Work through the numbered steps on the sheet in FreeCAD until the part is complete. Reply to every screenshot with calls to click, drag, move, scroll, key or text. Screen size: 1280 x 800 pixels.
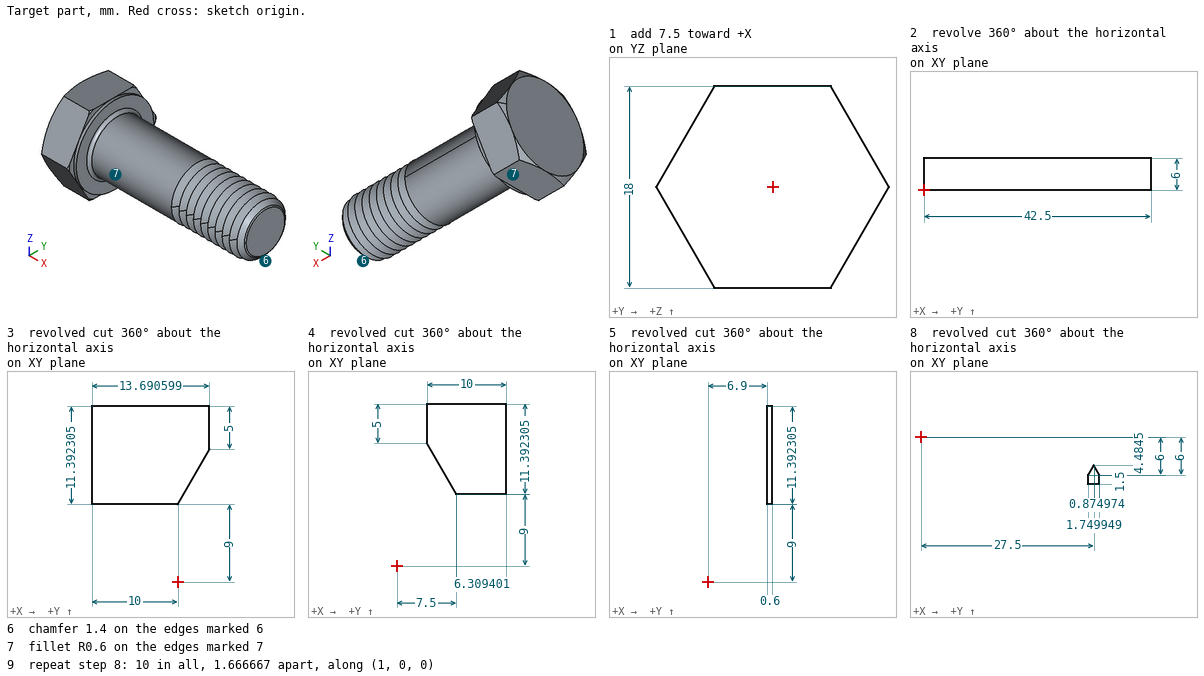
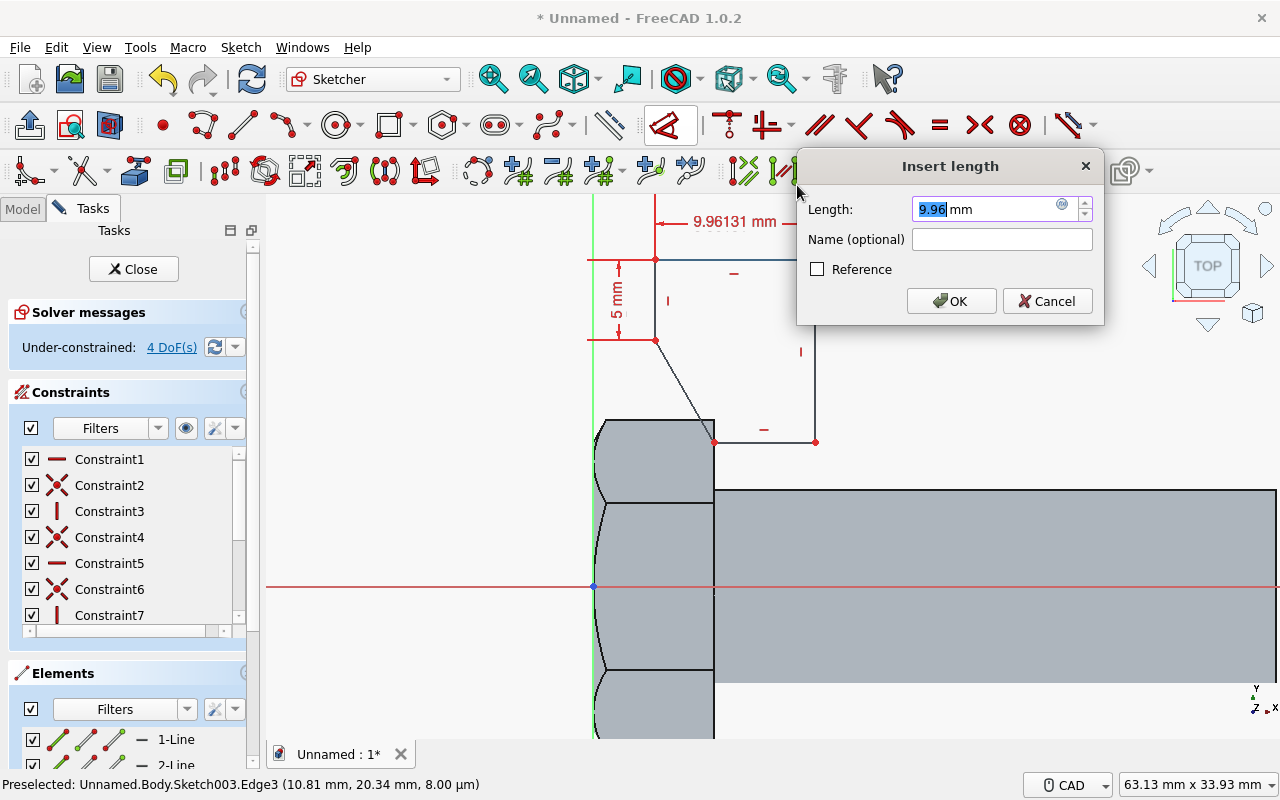
text(10)
key(Return)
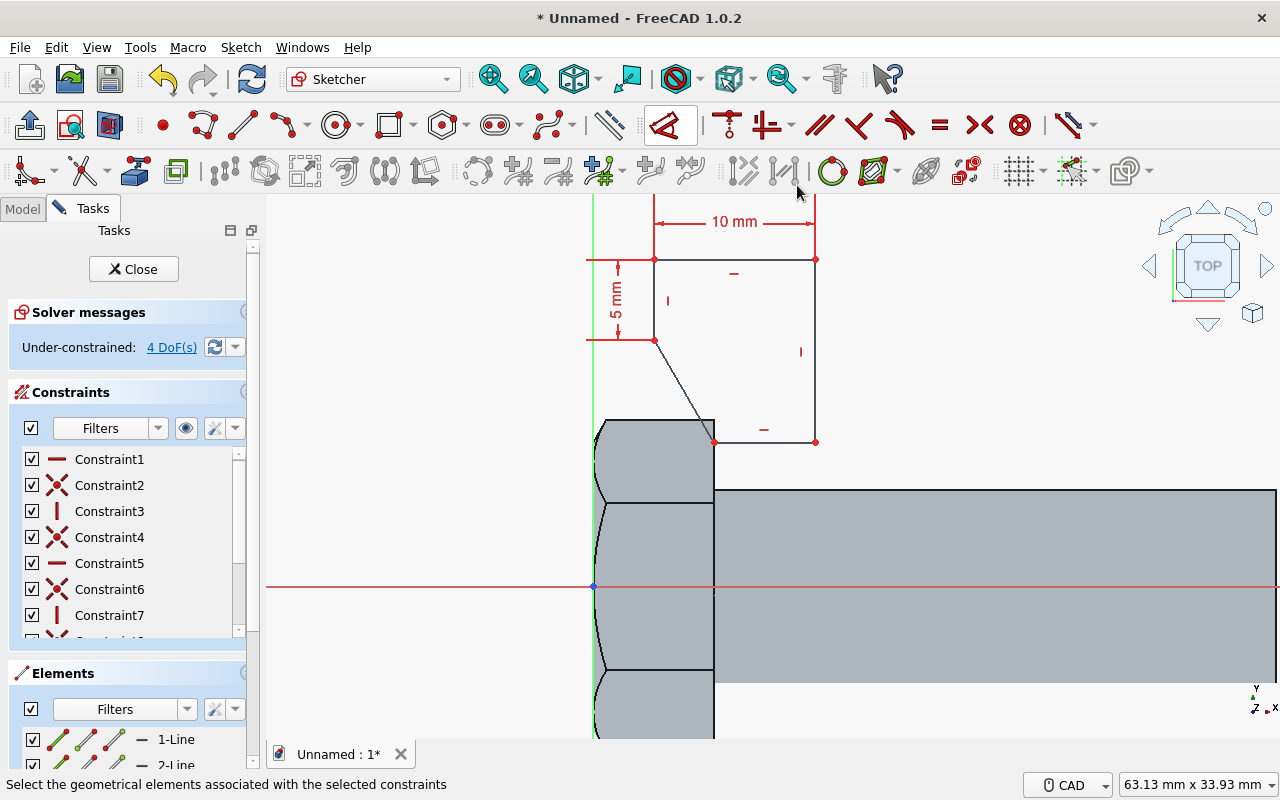
click(714, 443)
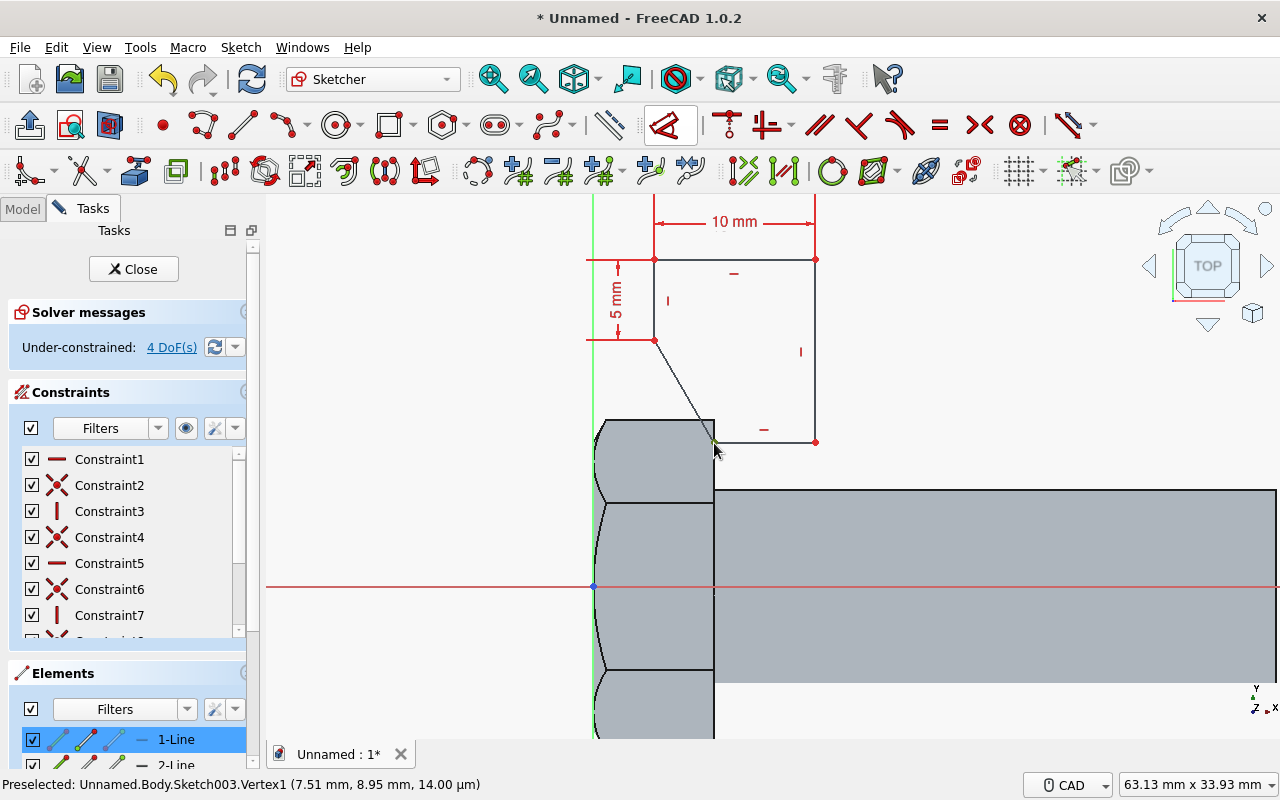
click(692, 126)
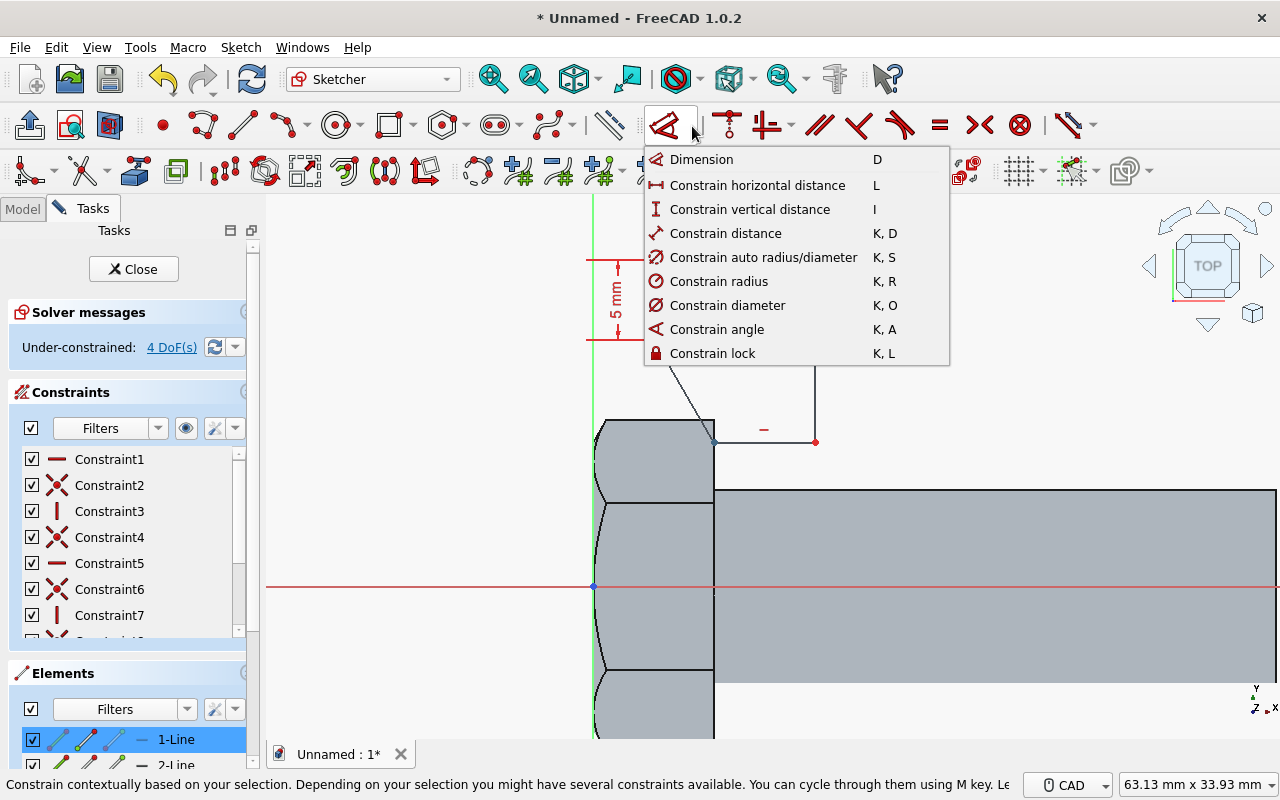
click(797, 209)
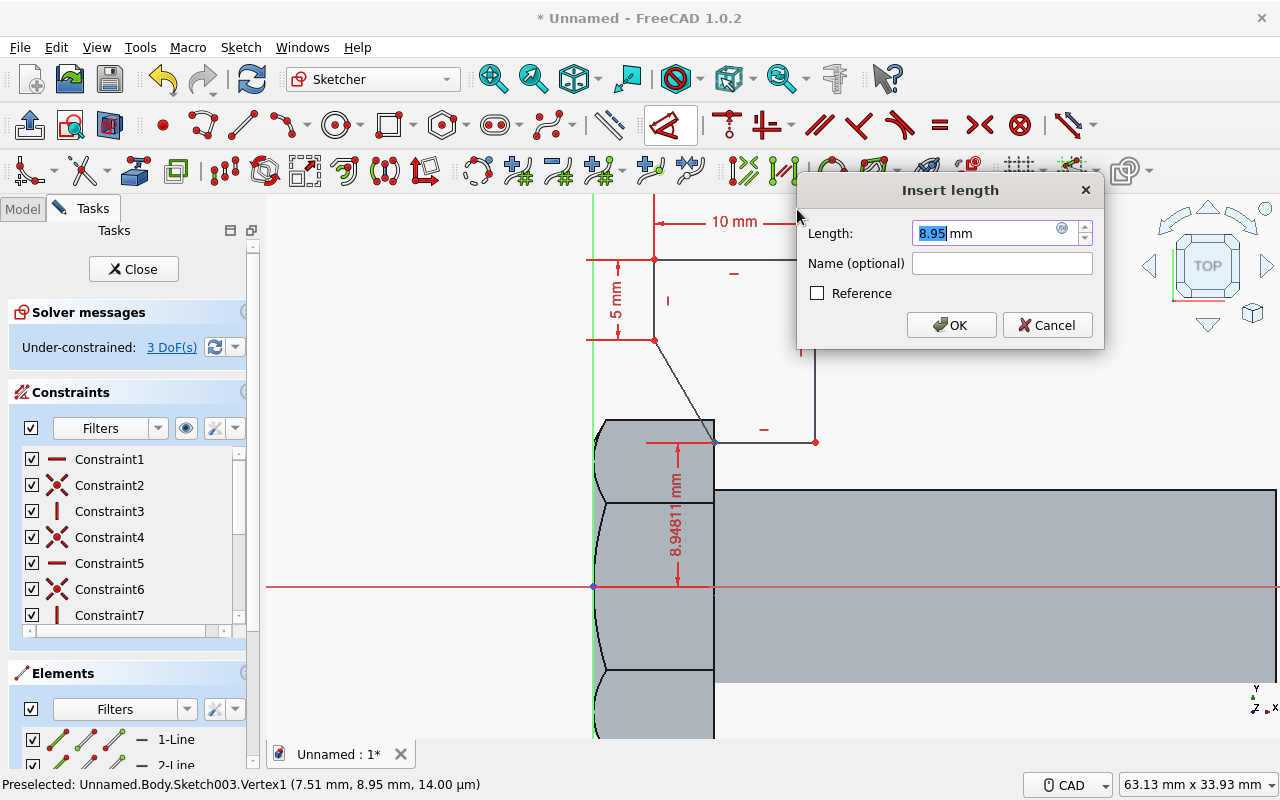
text(9)
key(Return)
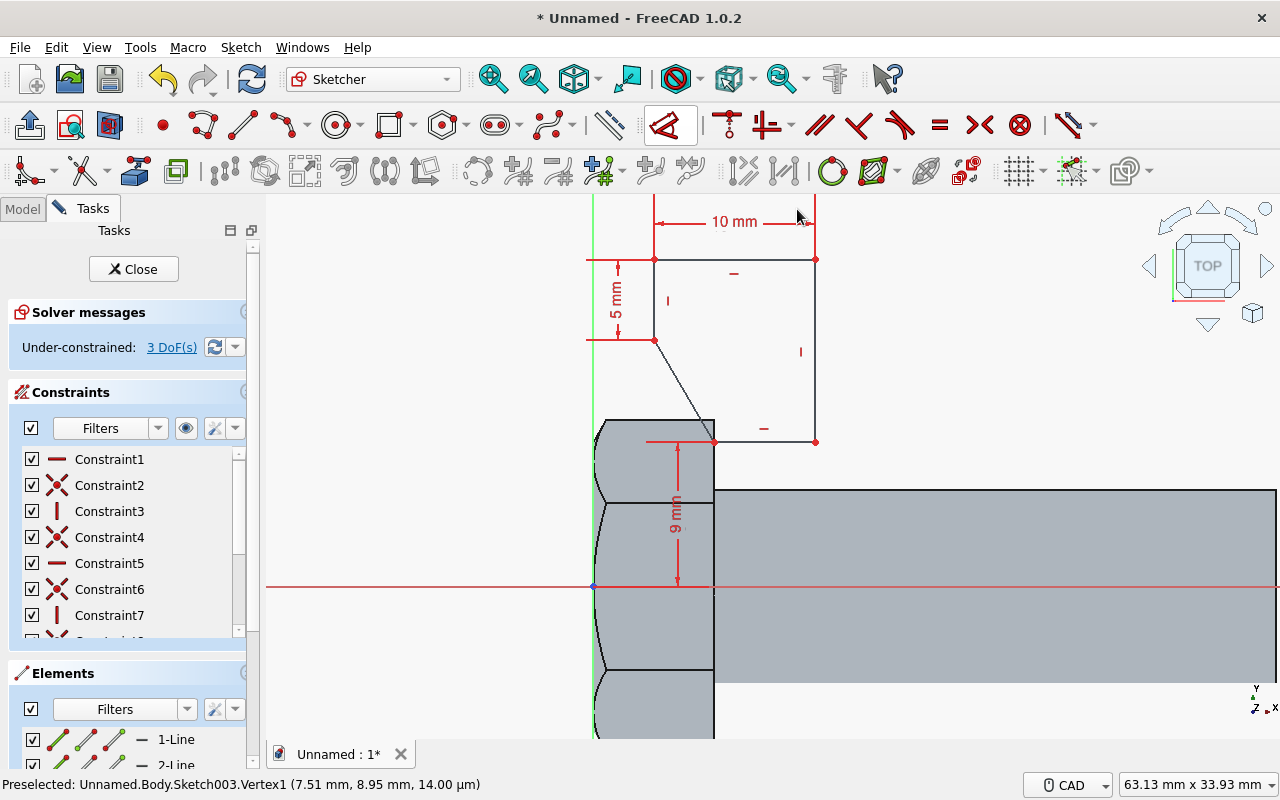
click(714, 442)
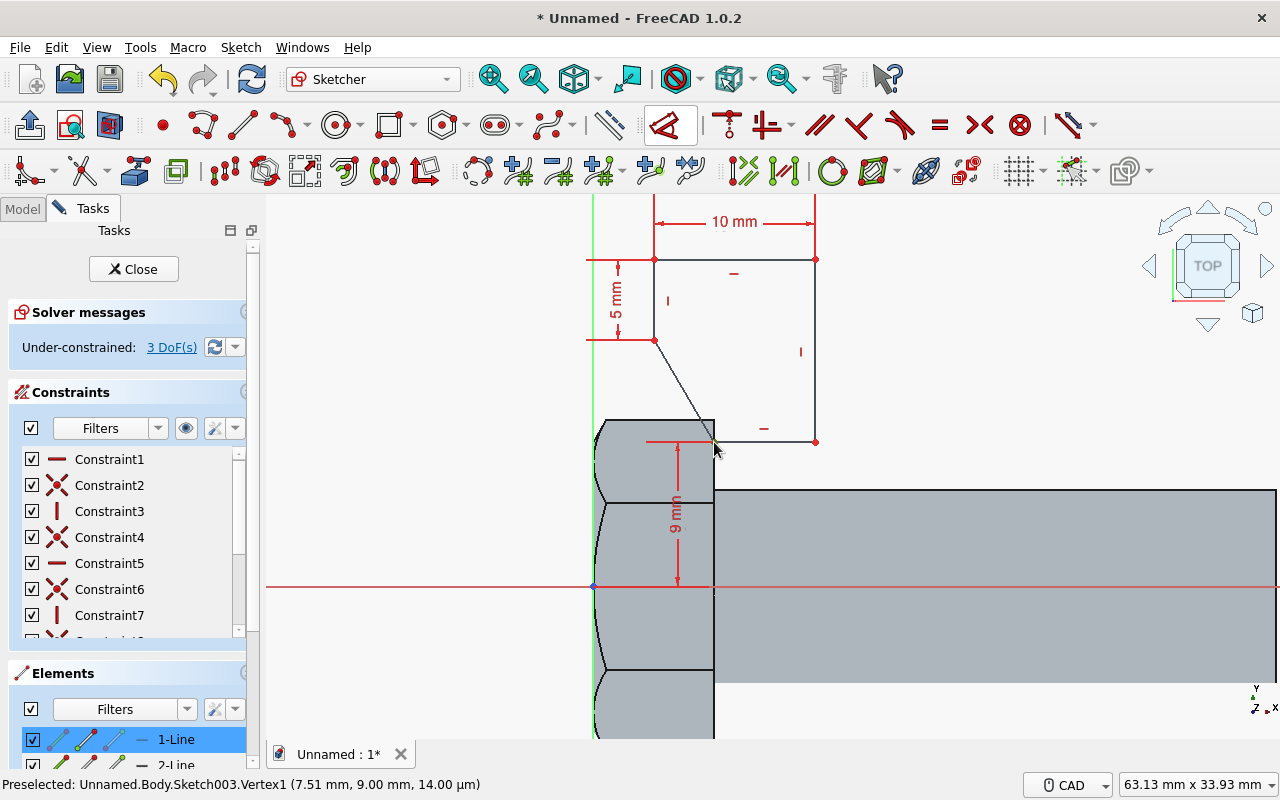
key(l)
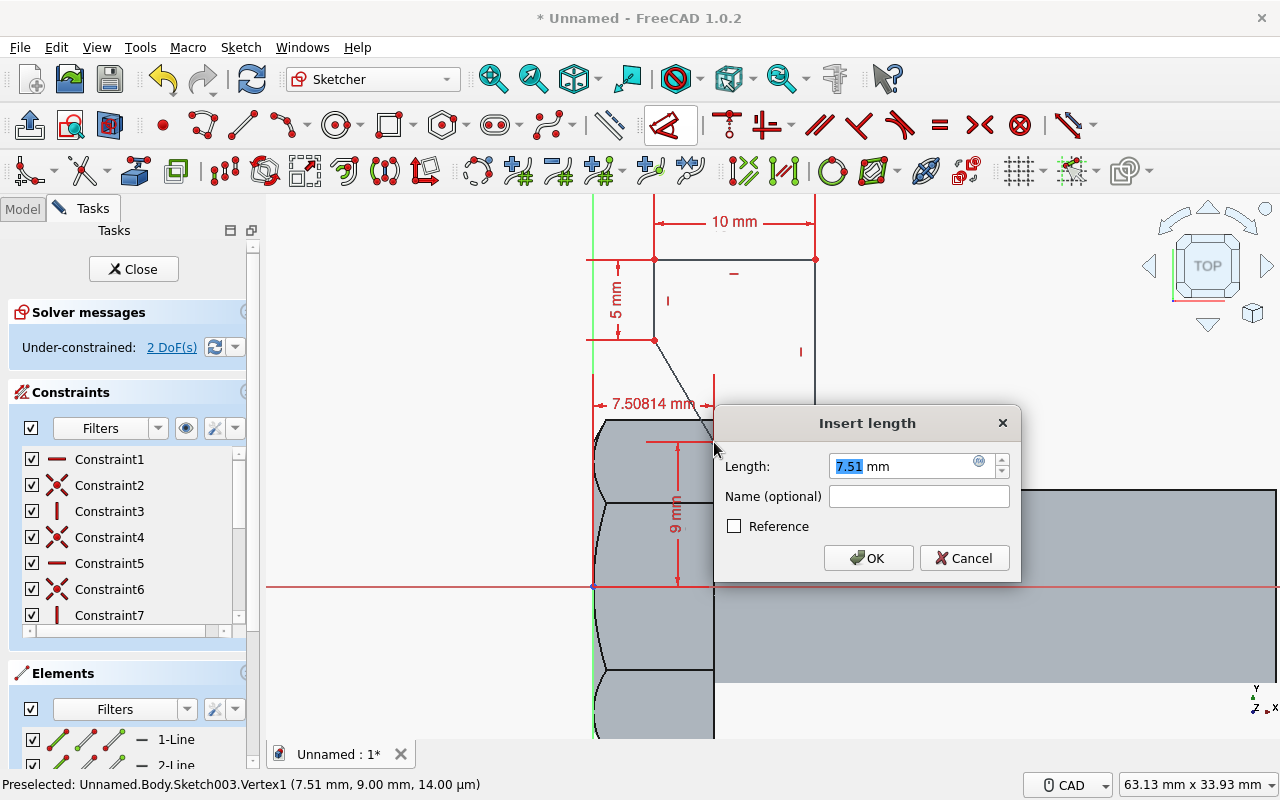
text(7.5)
key(Return)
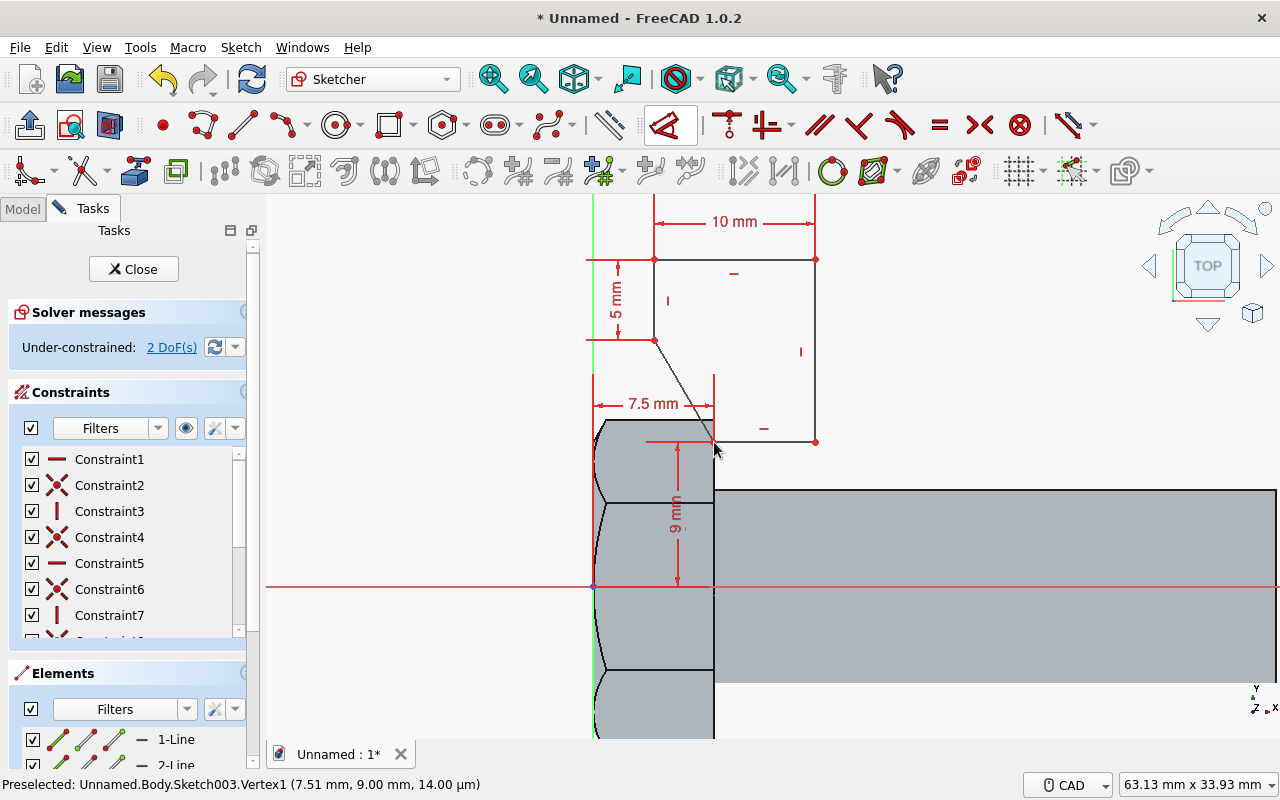
click(744, 442)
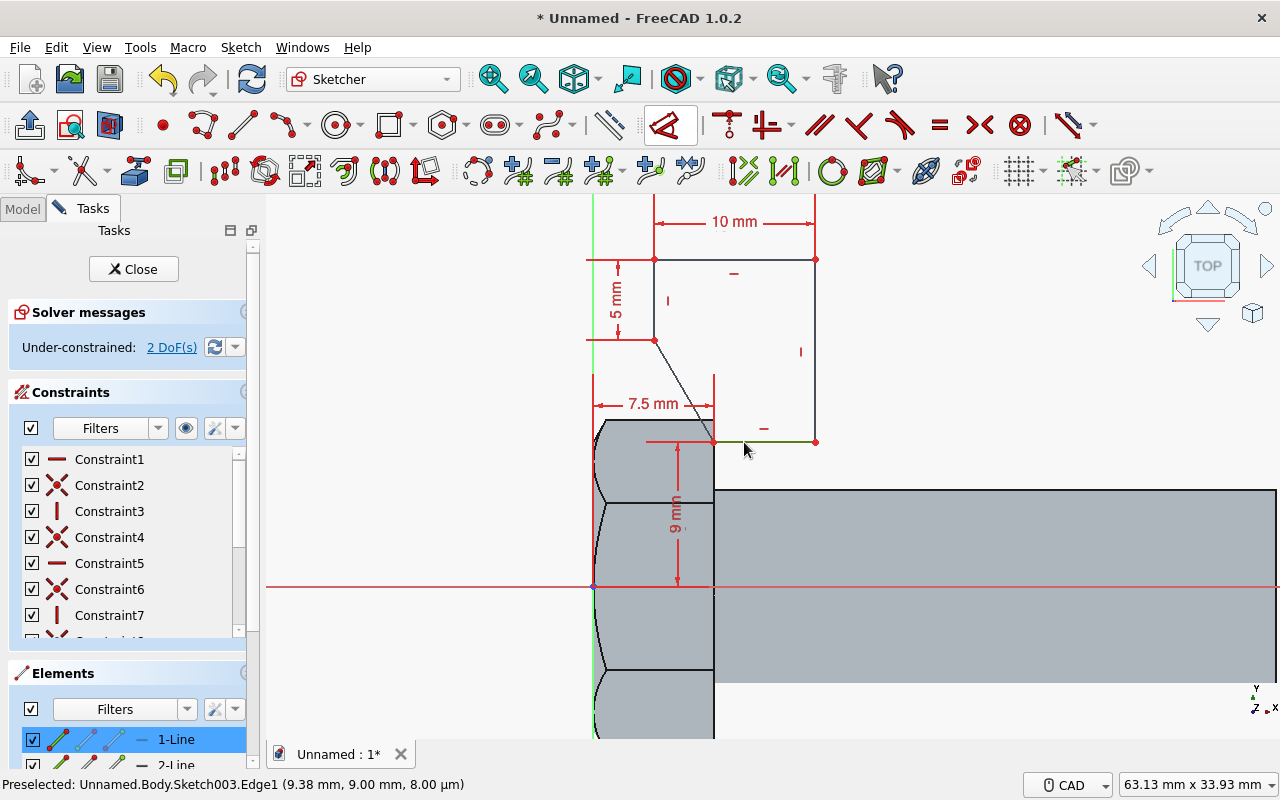
key(l)